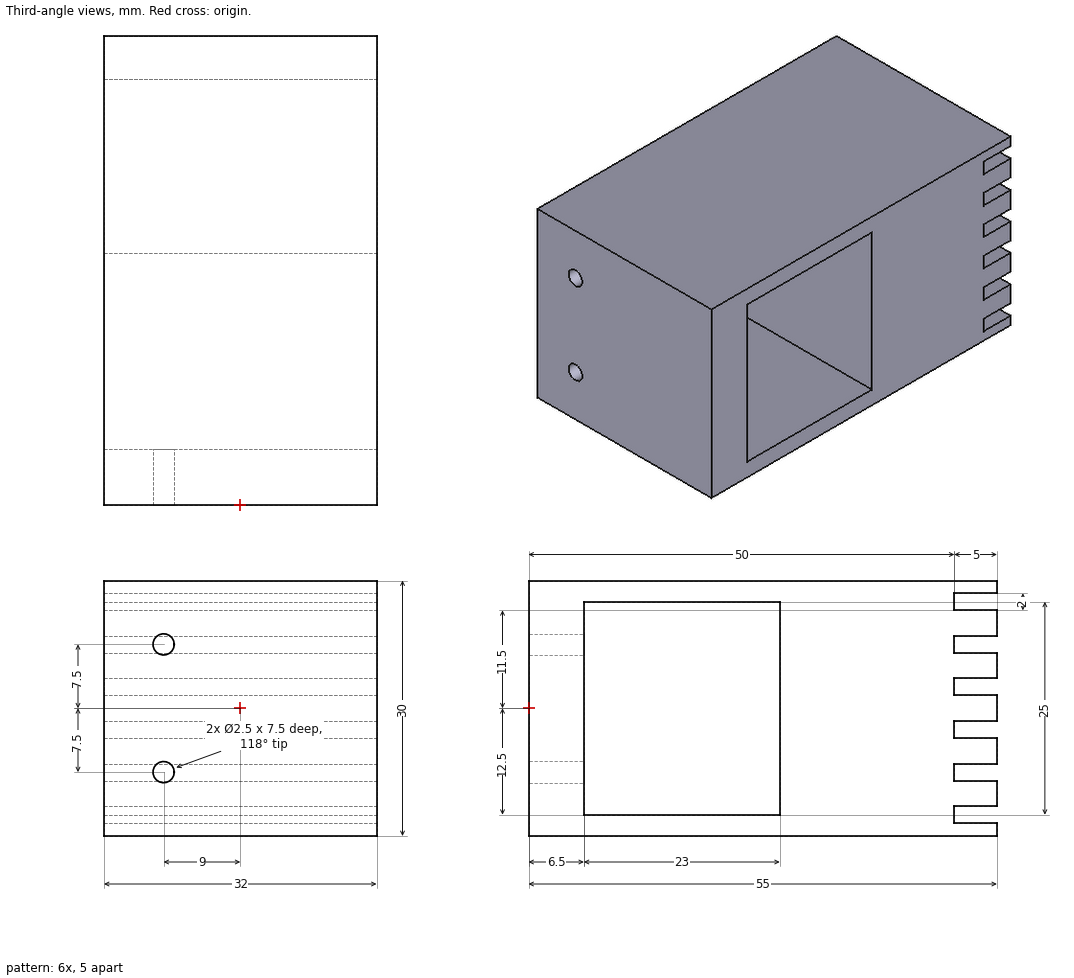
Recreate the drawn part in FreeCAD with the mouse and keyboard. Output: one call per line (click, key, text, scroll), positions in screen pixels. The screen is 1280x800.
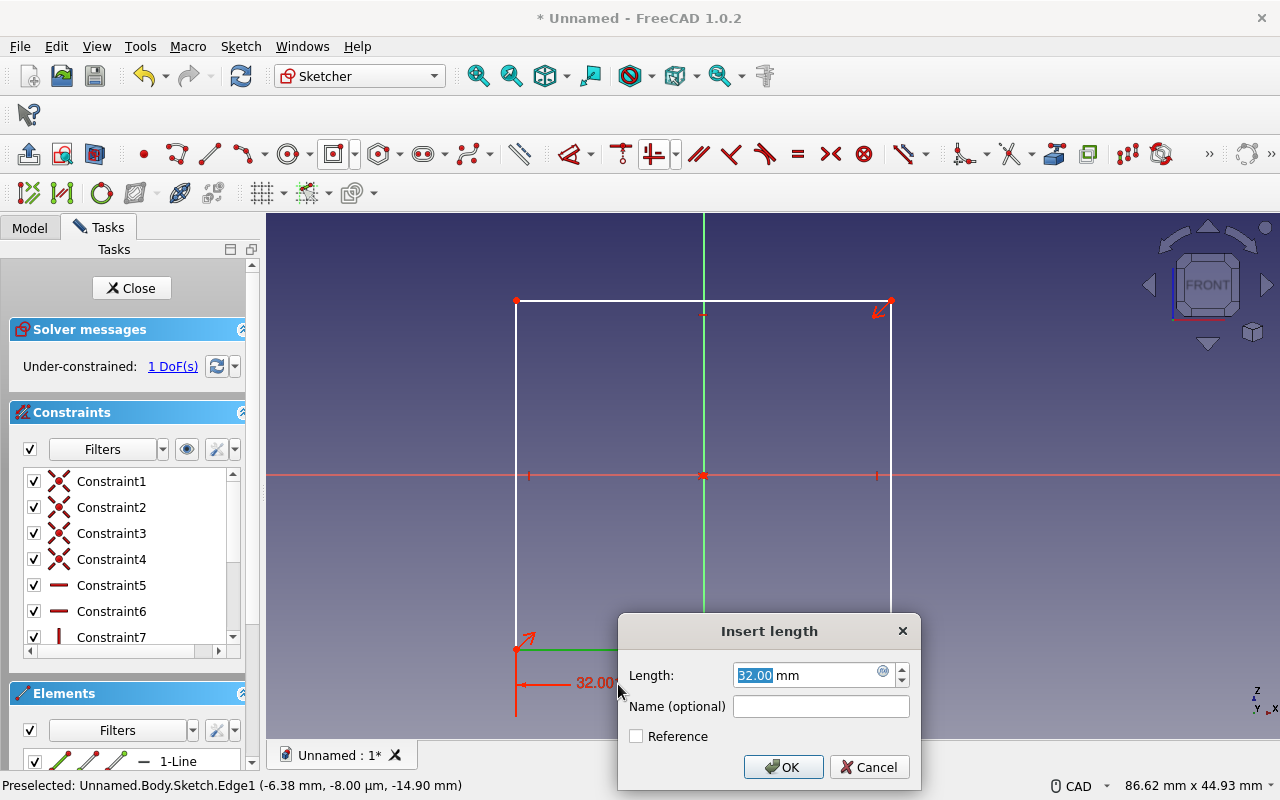
text(32)
key(Return)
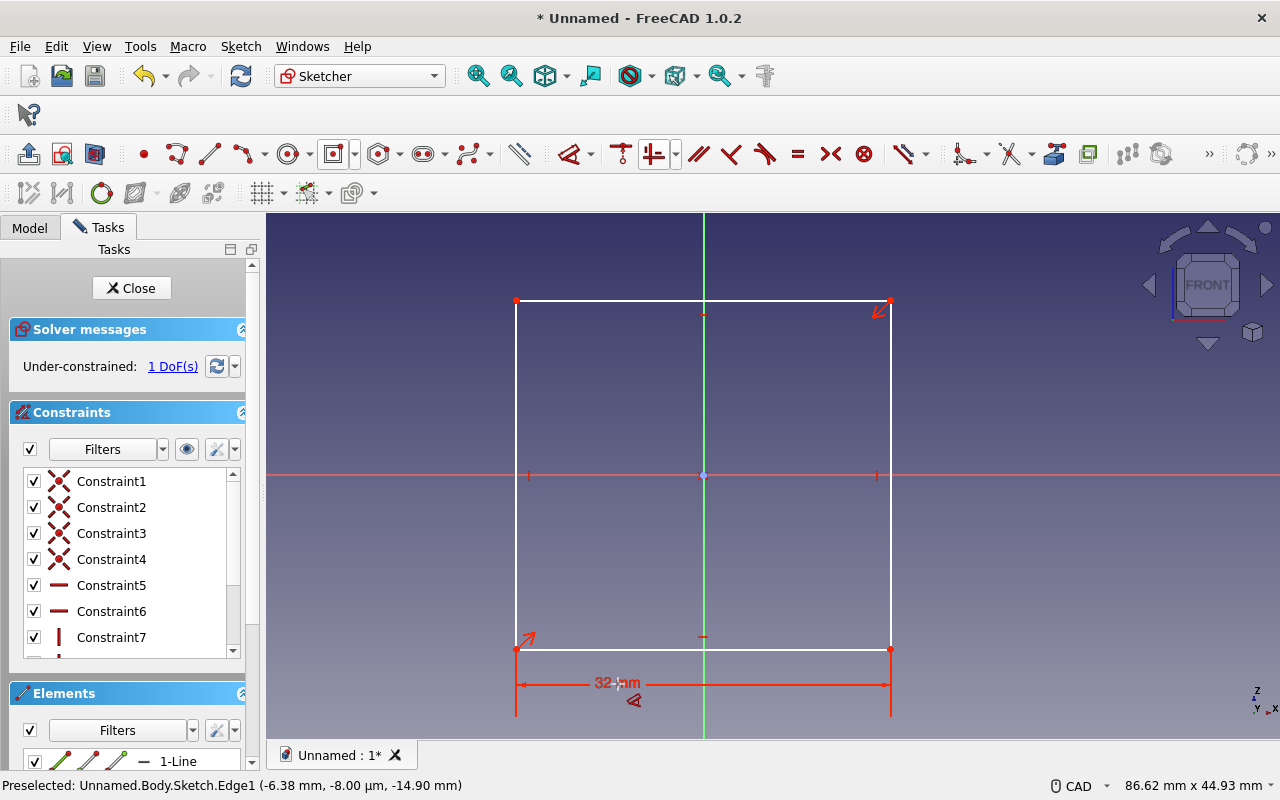
click(891, 545)
click(925, 395)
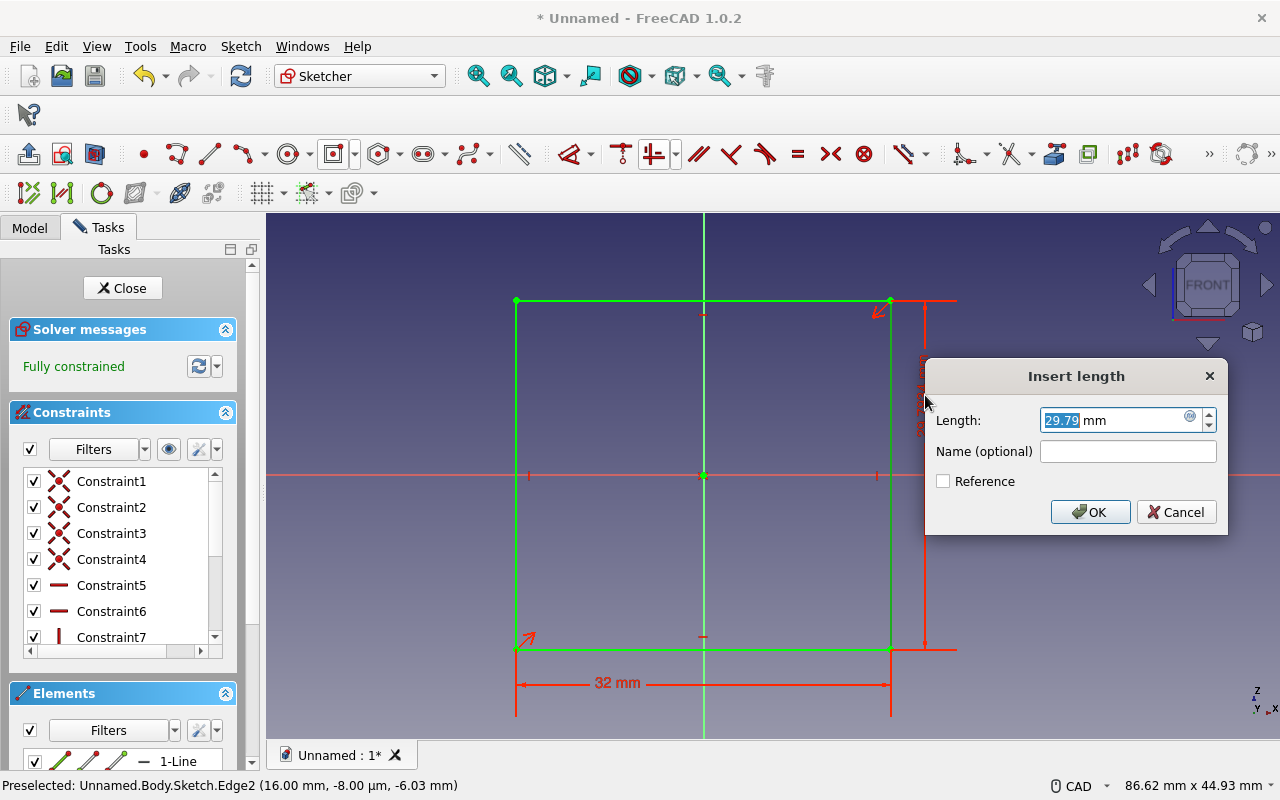
text(30)
key(Return)
key(Escape)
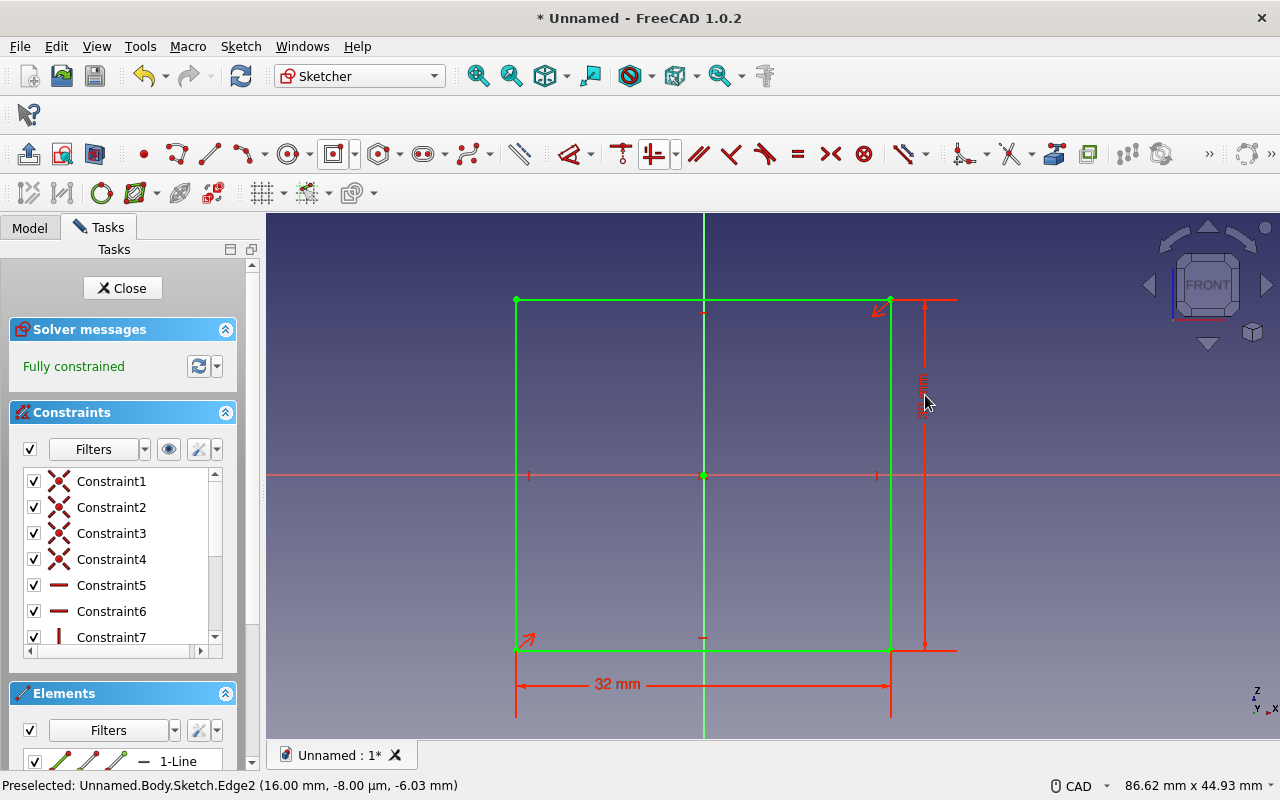
click(123, 288)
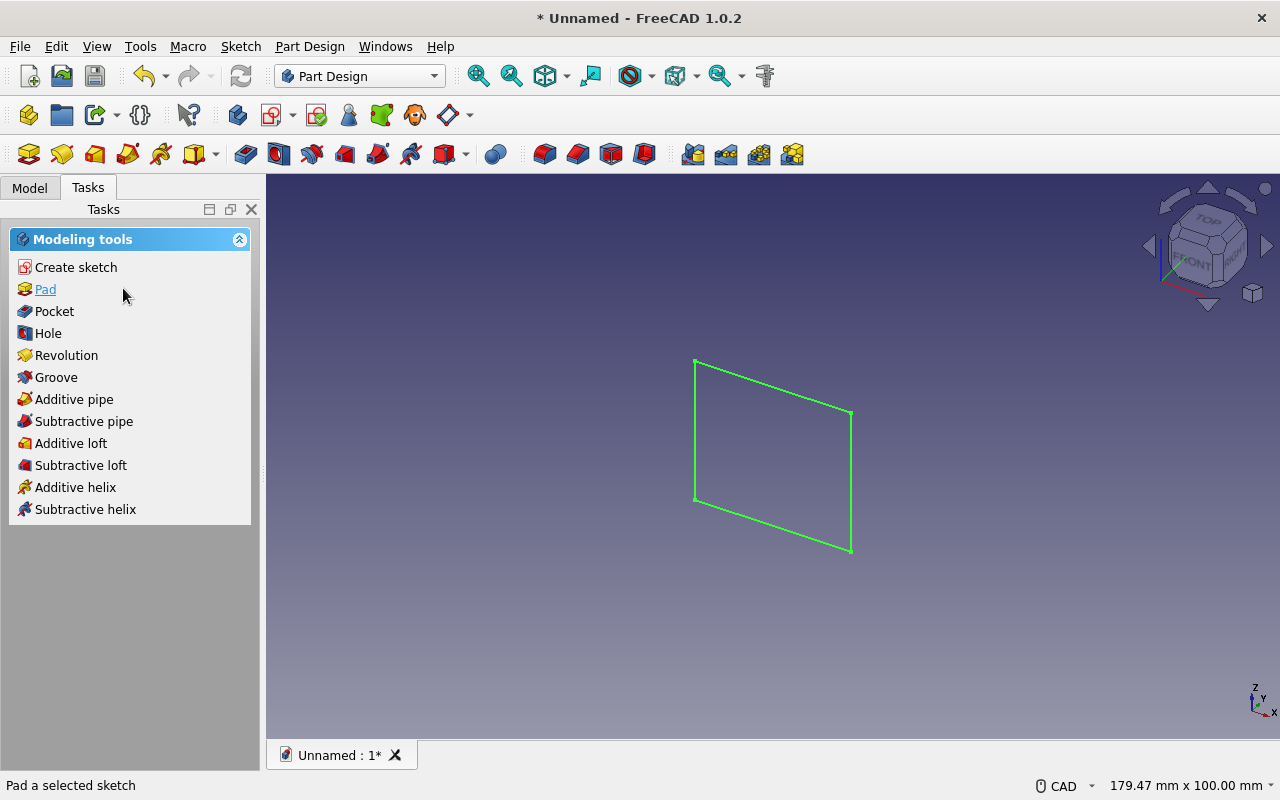
click(29, 154)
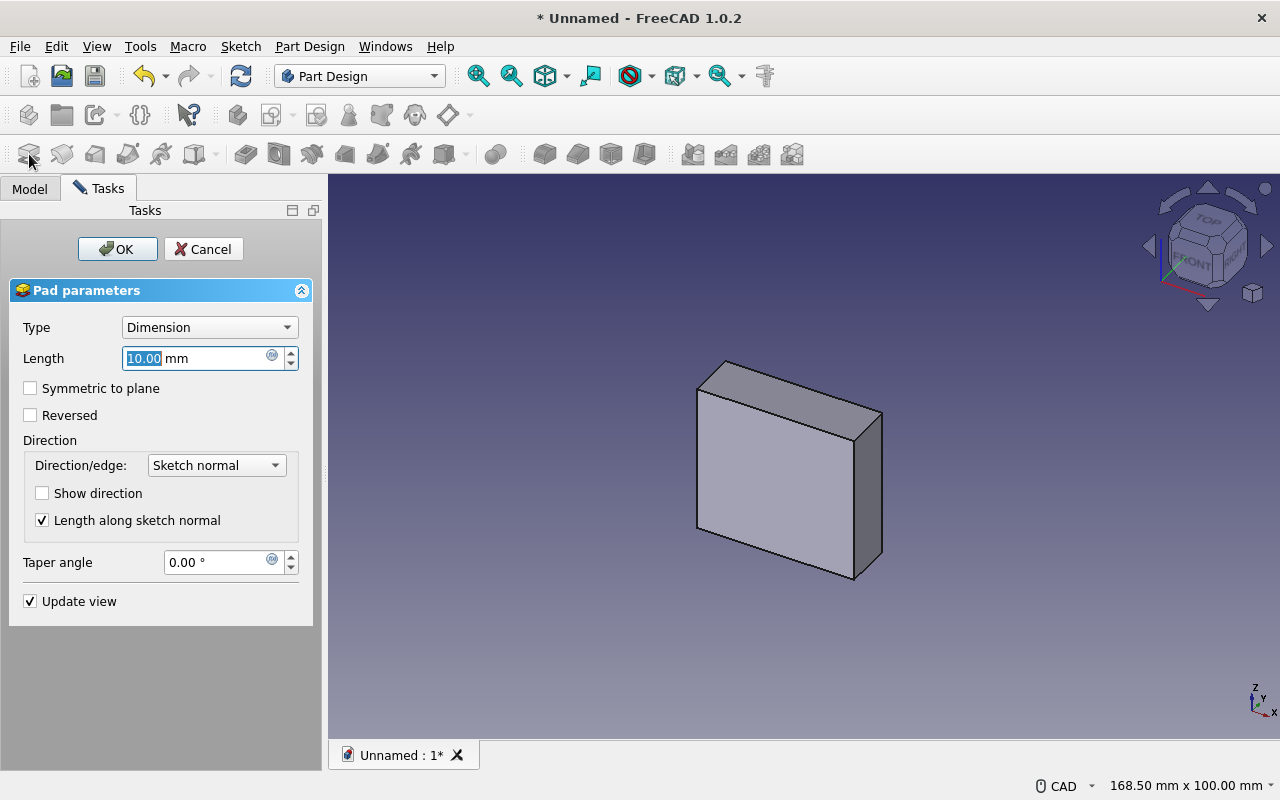
text(55)
key(Tab)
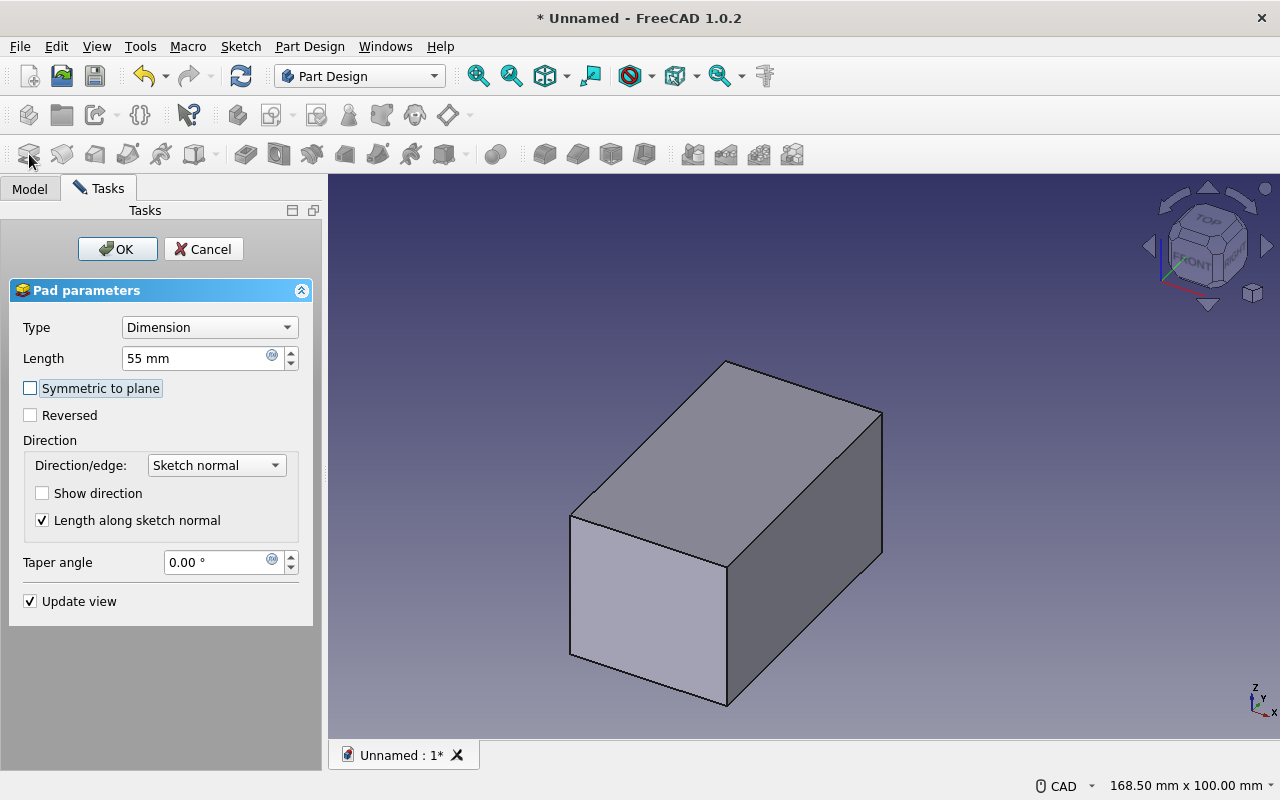
click(31, 415)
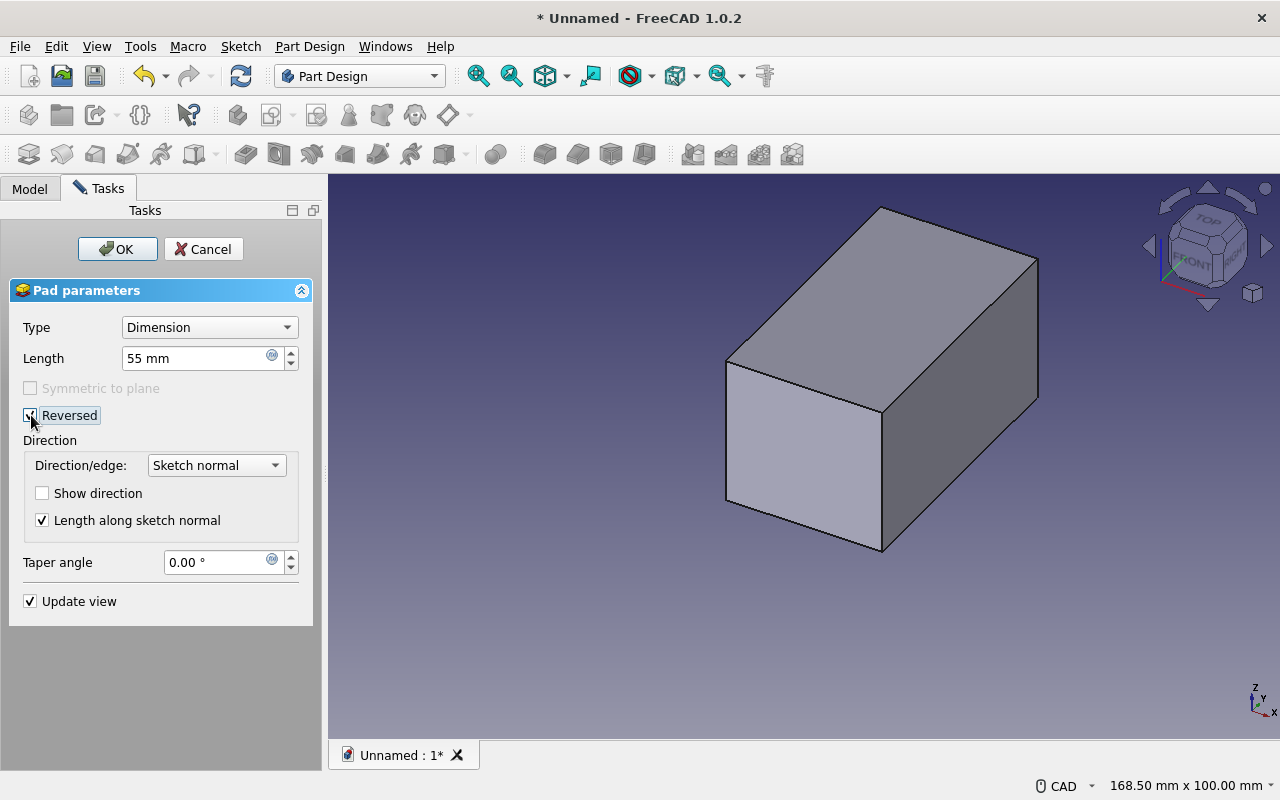
click(118, 249)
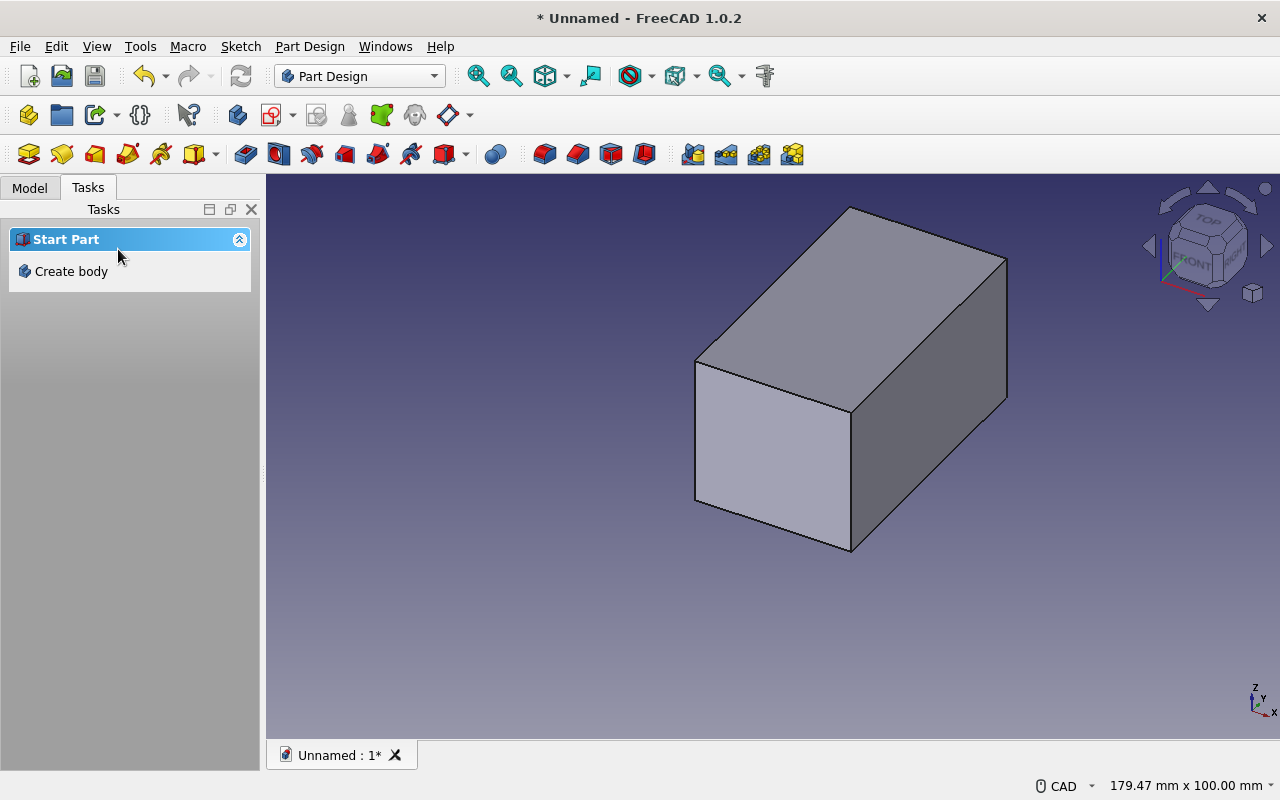
click(270, 116)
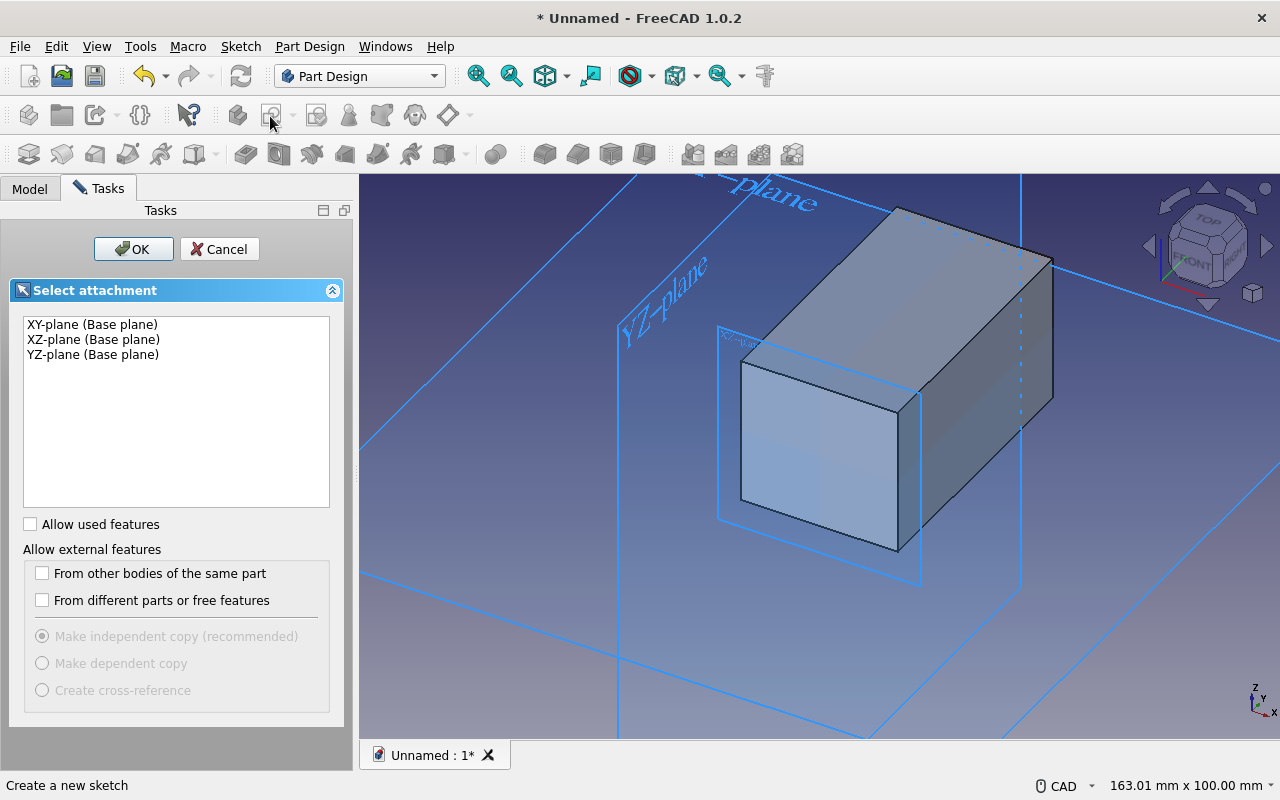
click(84, 340)